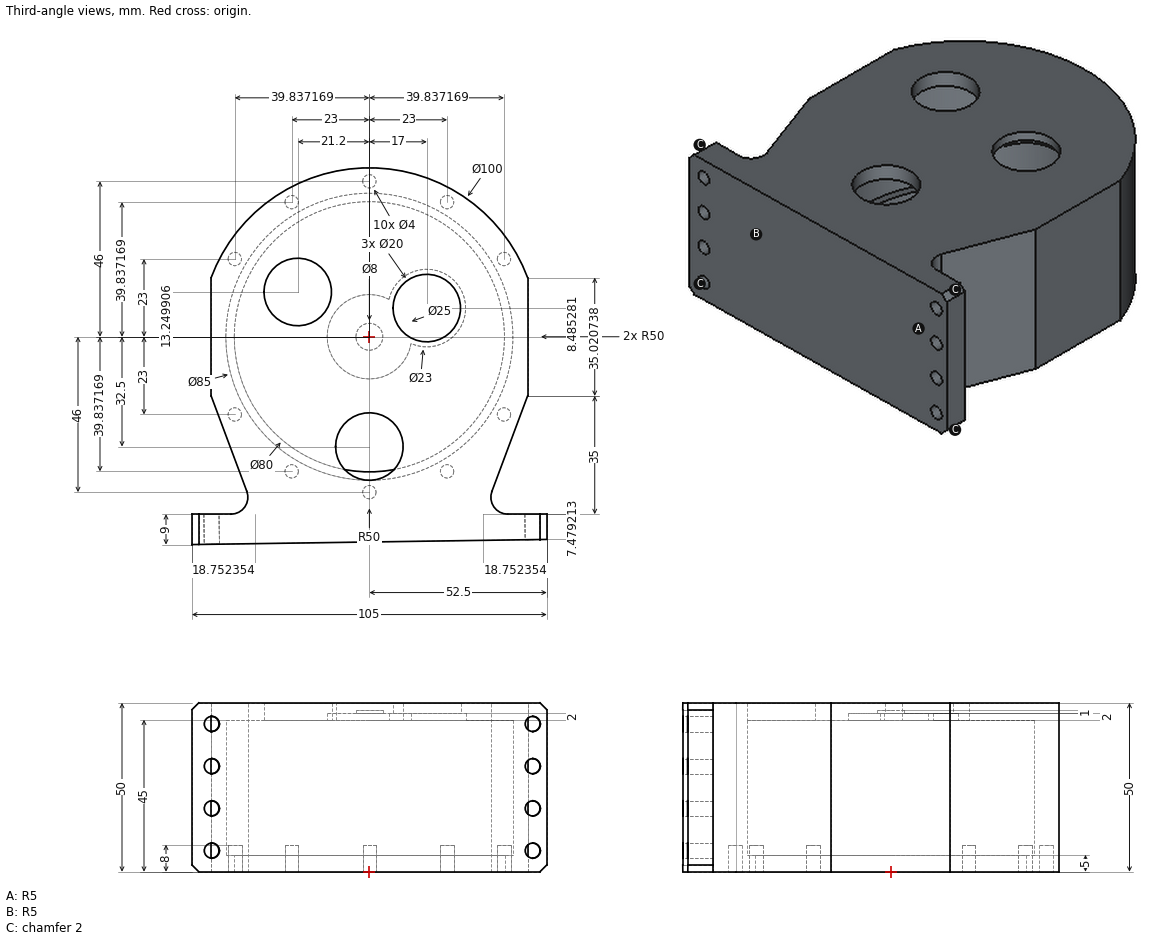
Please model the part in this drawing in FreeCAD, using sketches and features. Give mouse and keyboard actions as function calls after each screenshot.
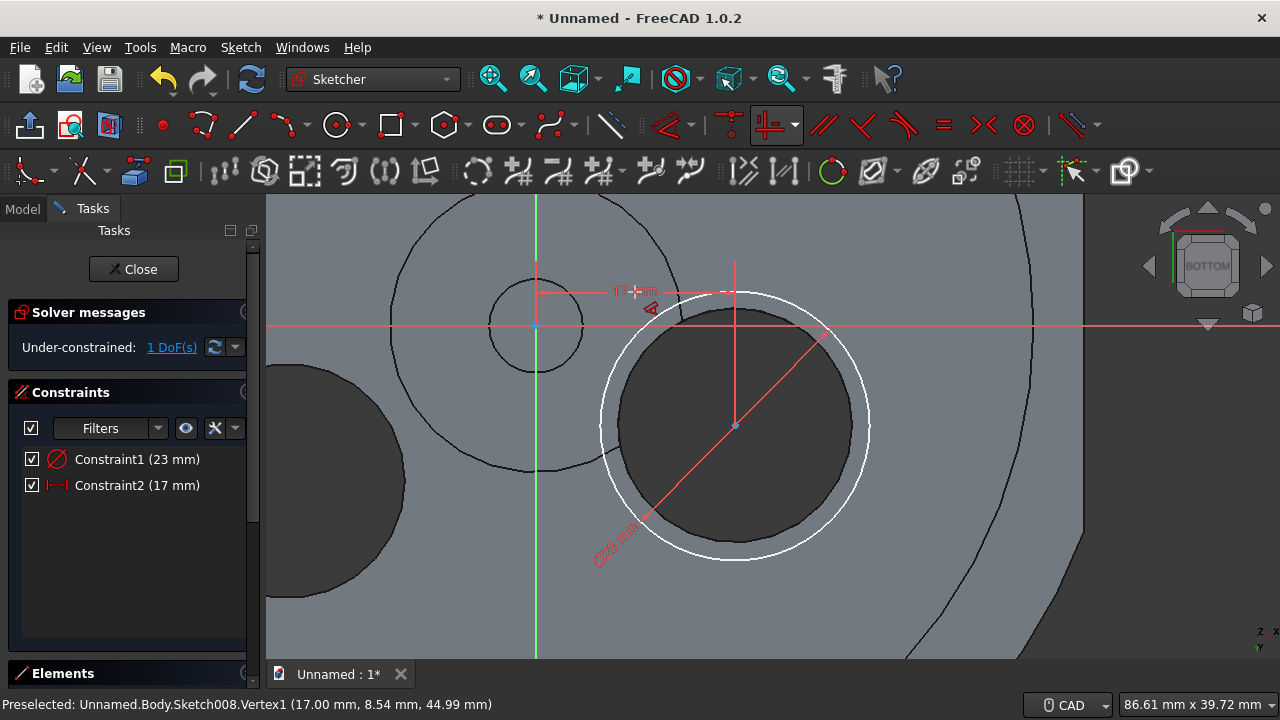
click(735, 426)
click(502, 376)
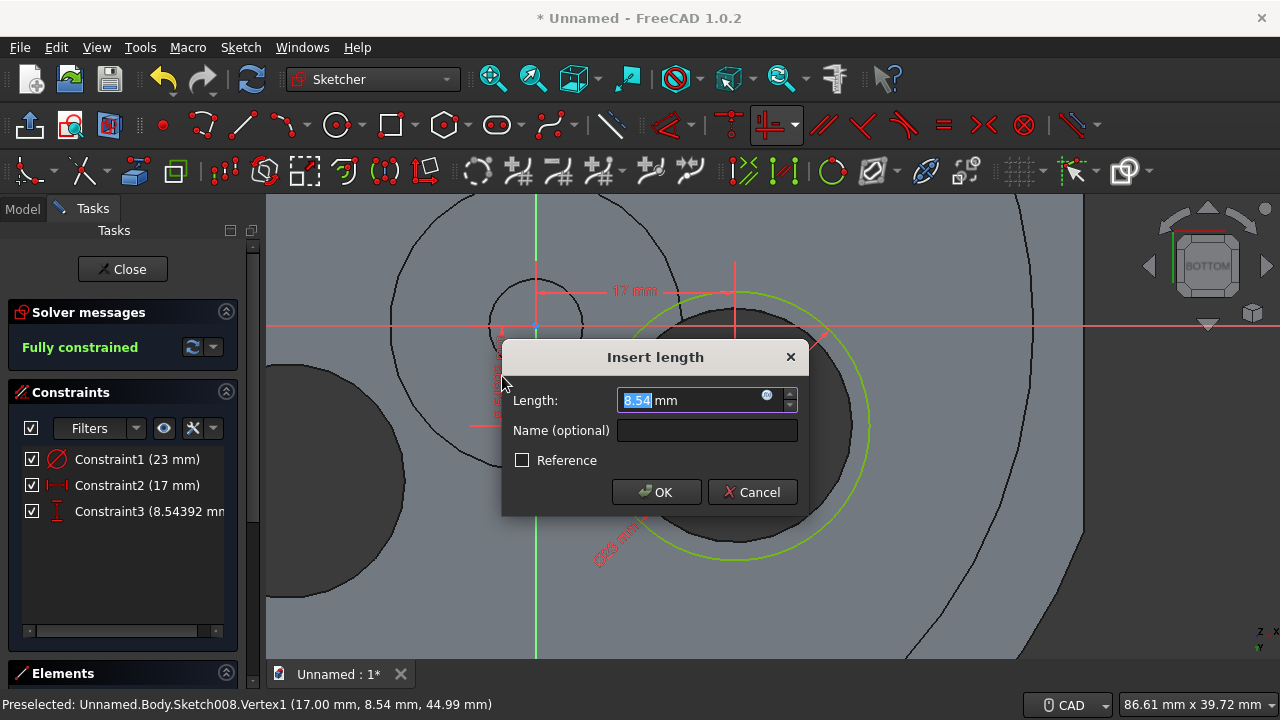
text(8.485281)
key(Return)
key(Escape)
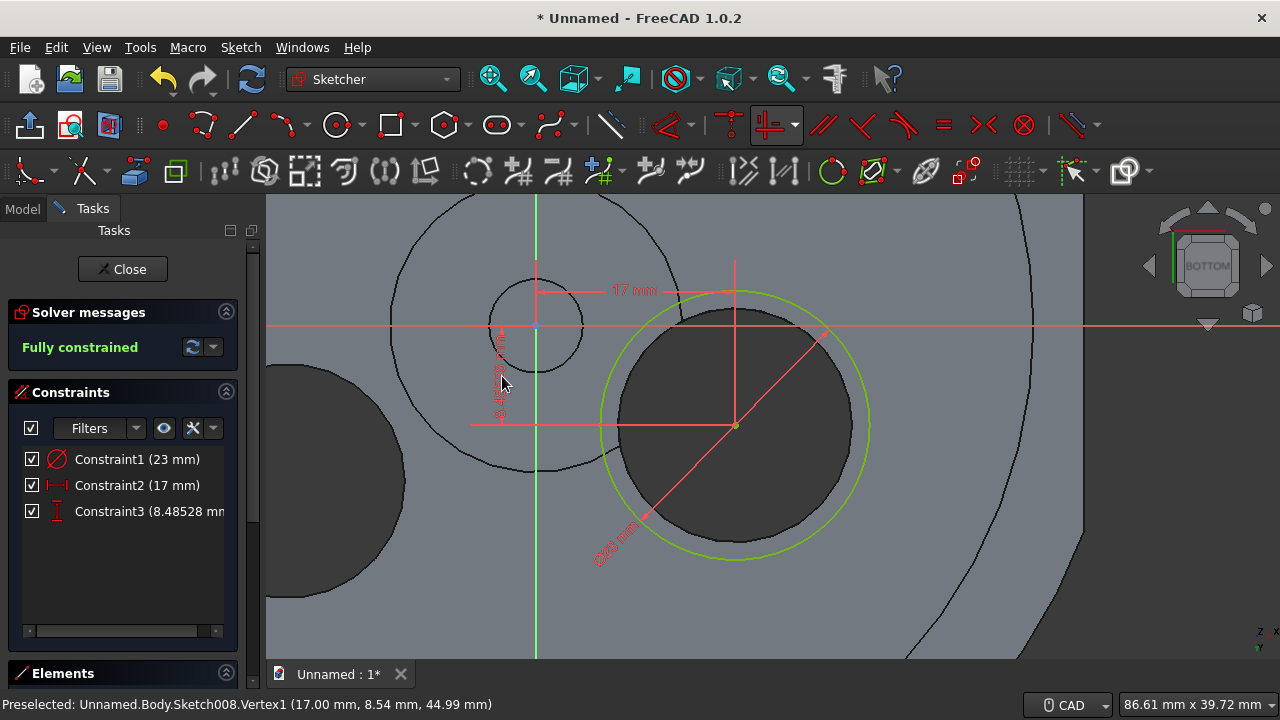
click(123, 269)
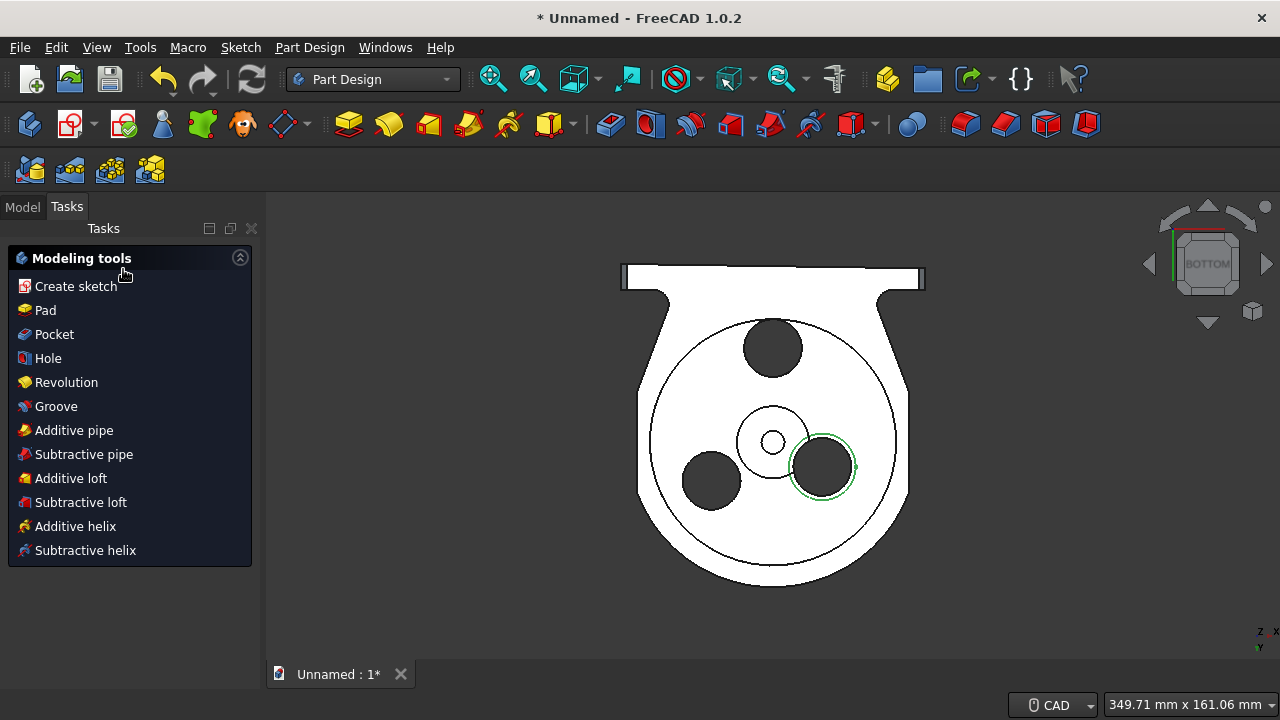
click(612, 124)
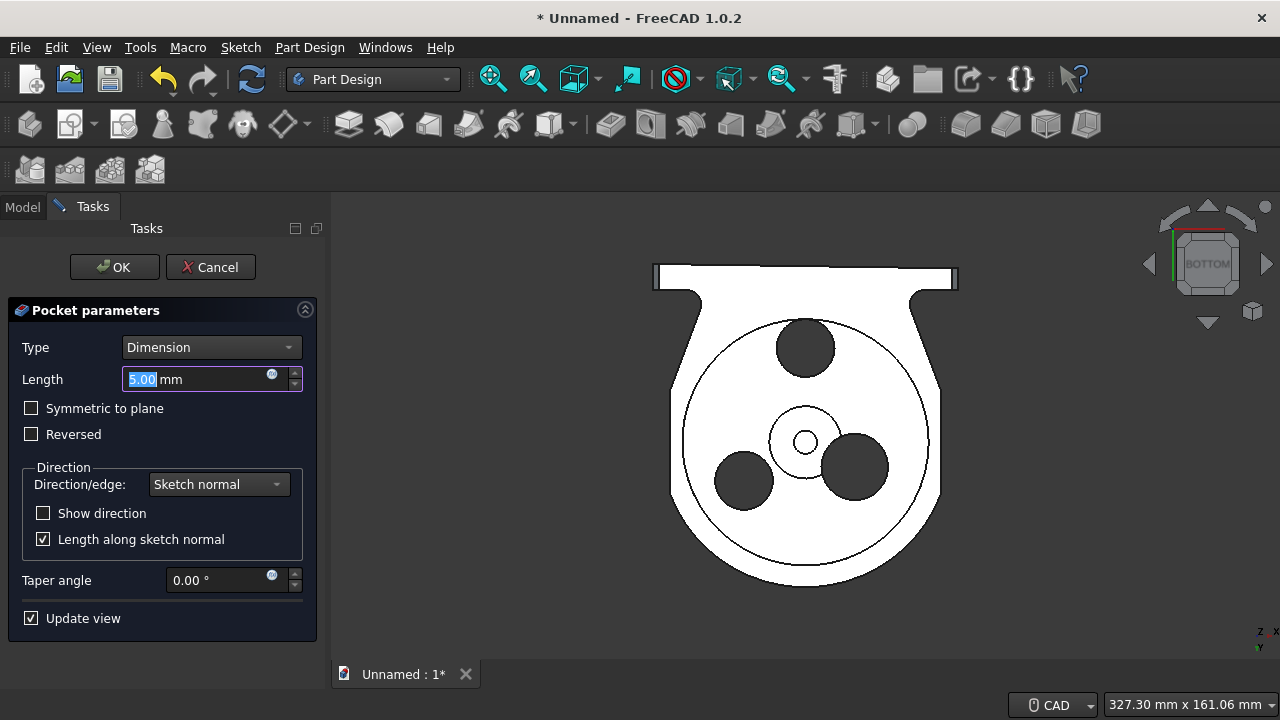
text(2)
key(Tab)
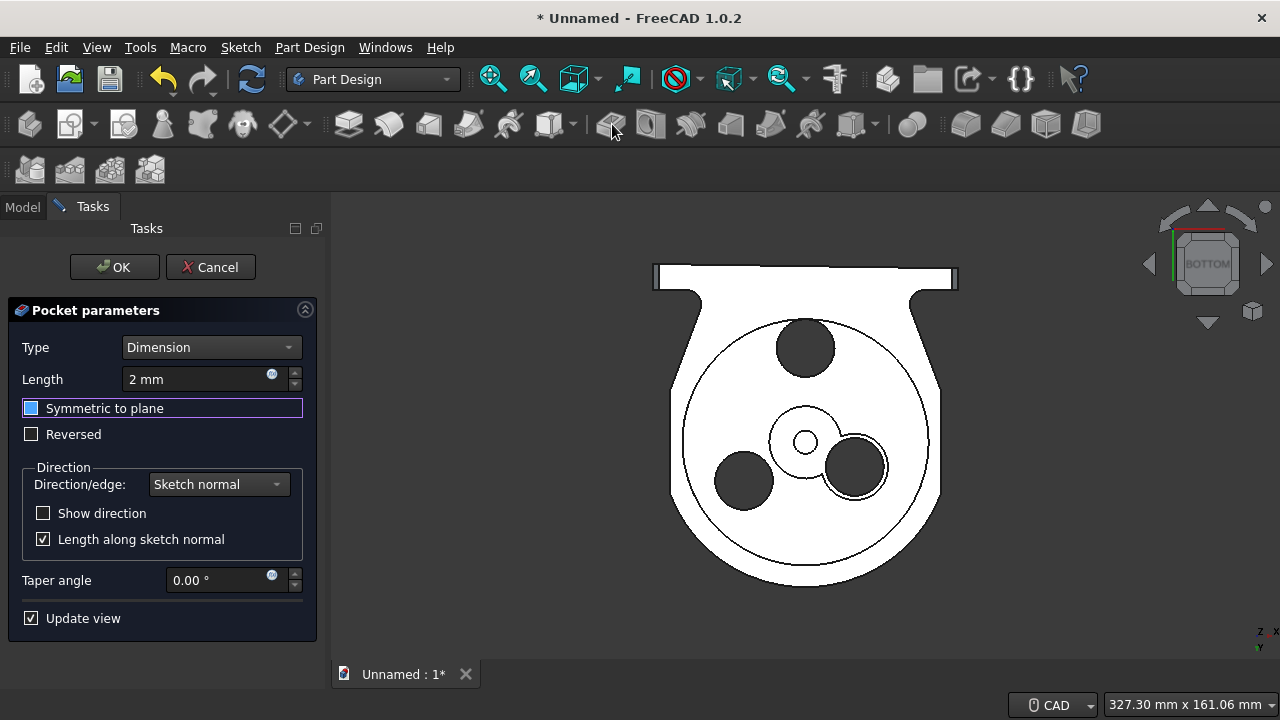
click(115, 267)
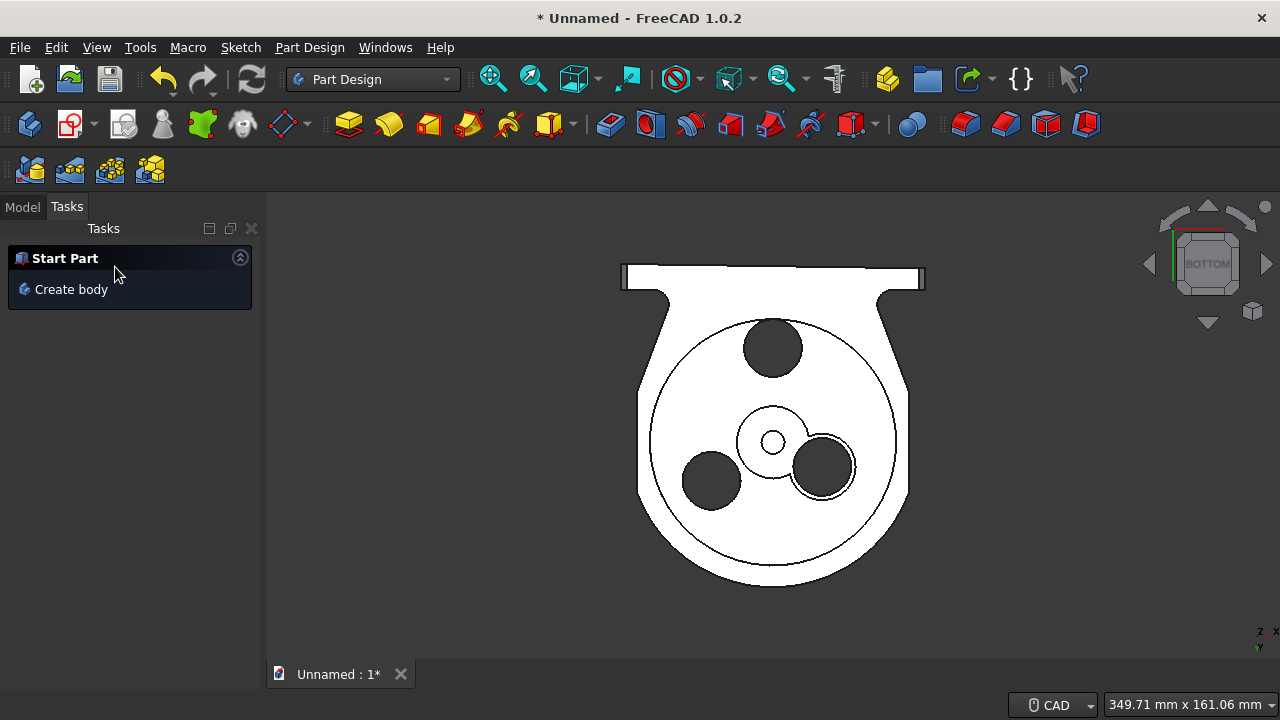
click(70, 124)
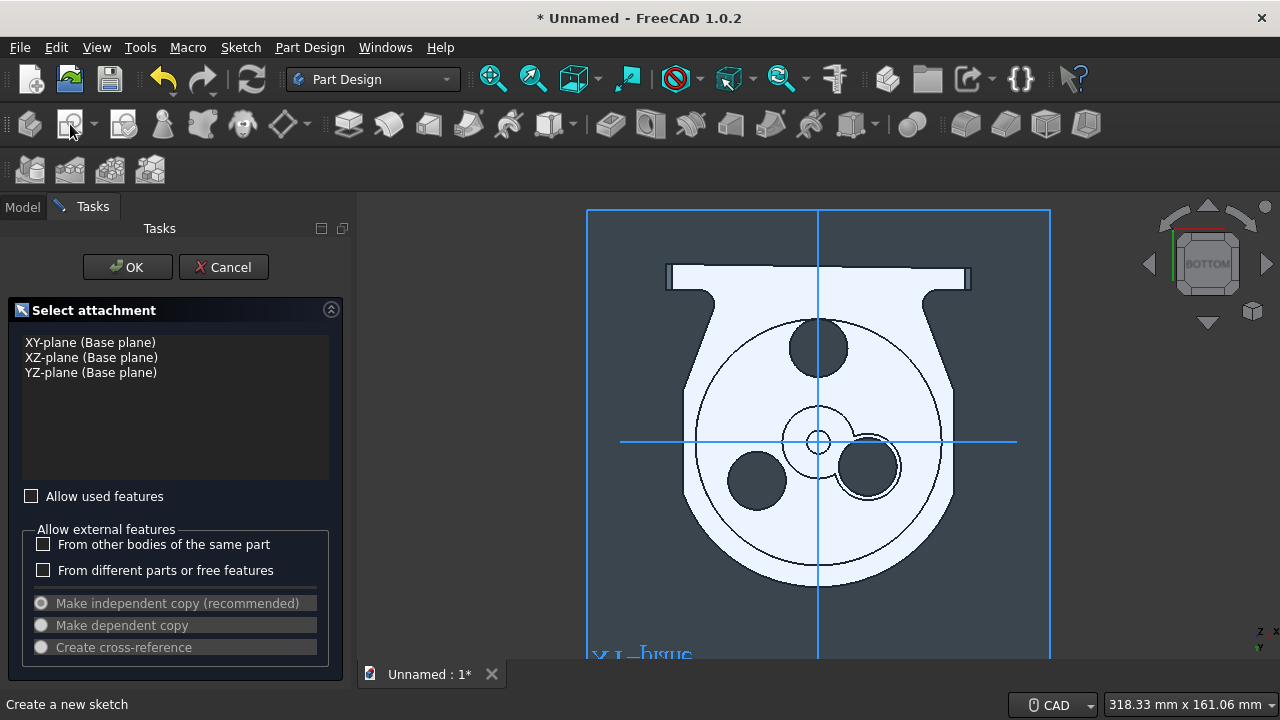
click(82, 342)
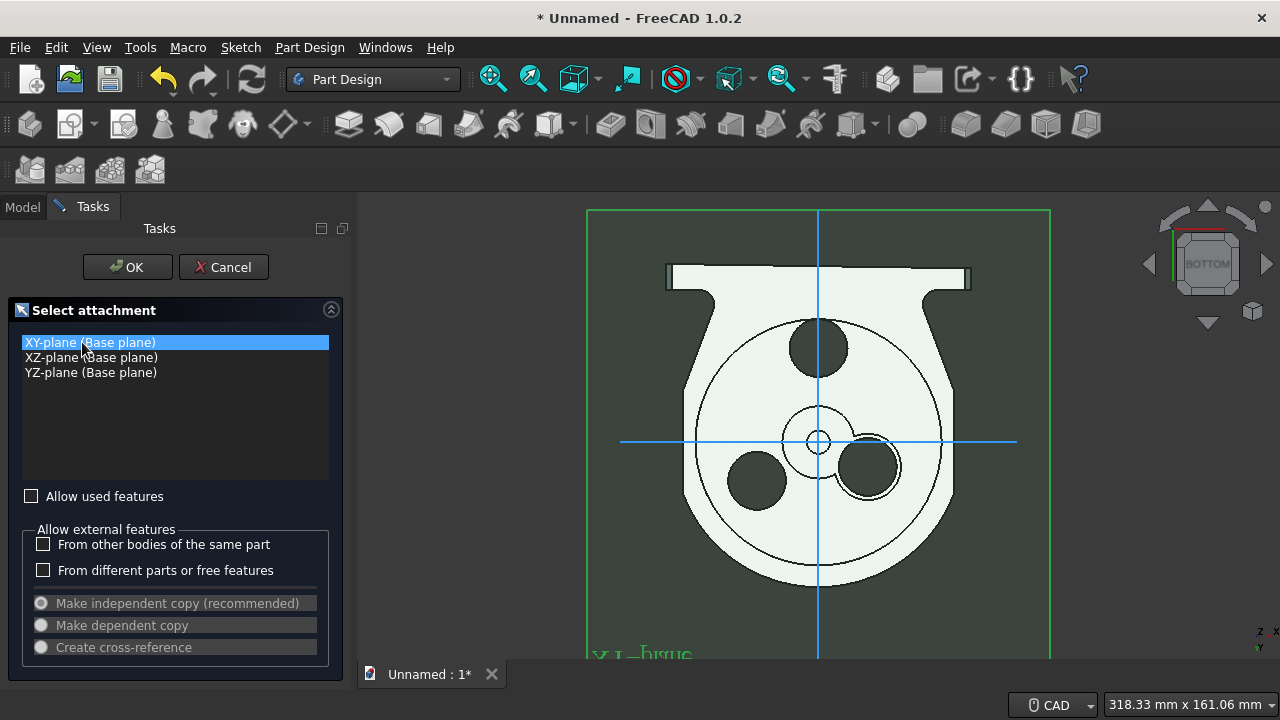
click(128, 267)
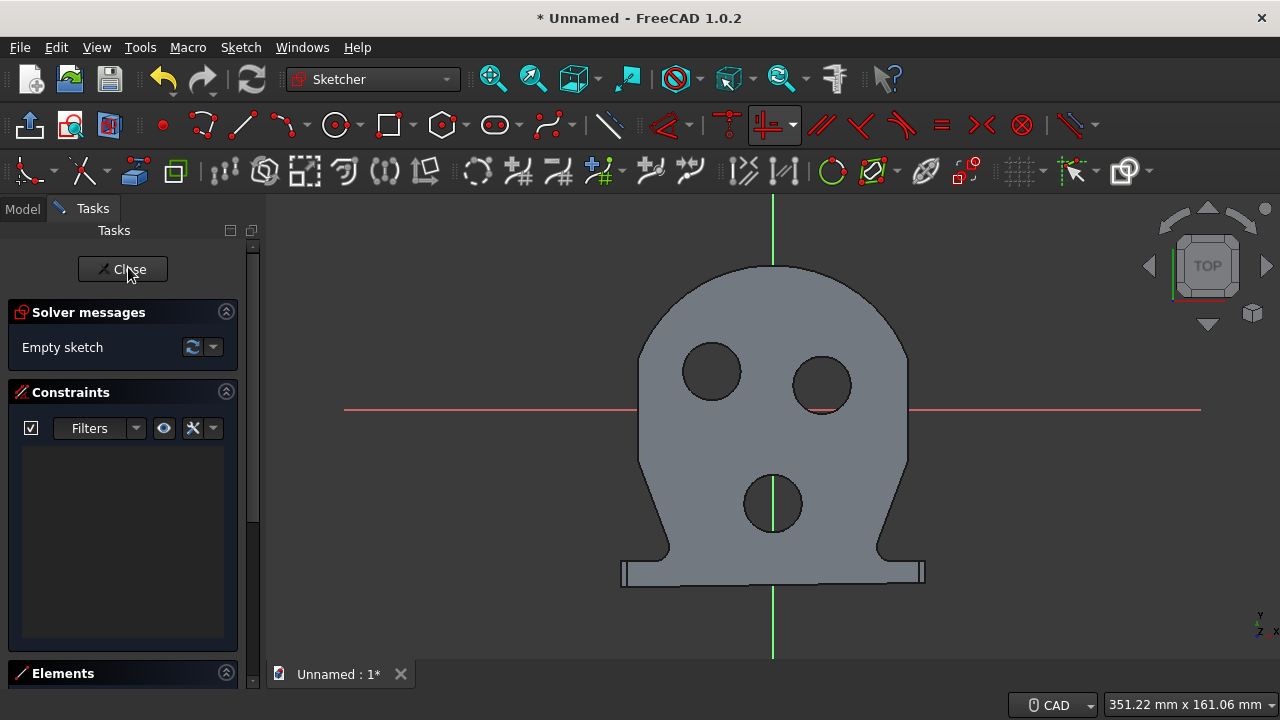
key(q)
key(s)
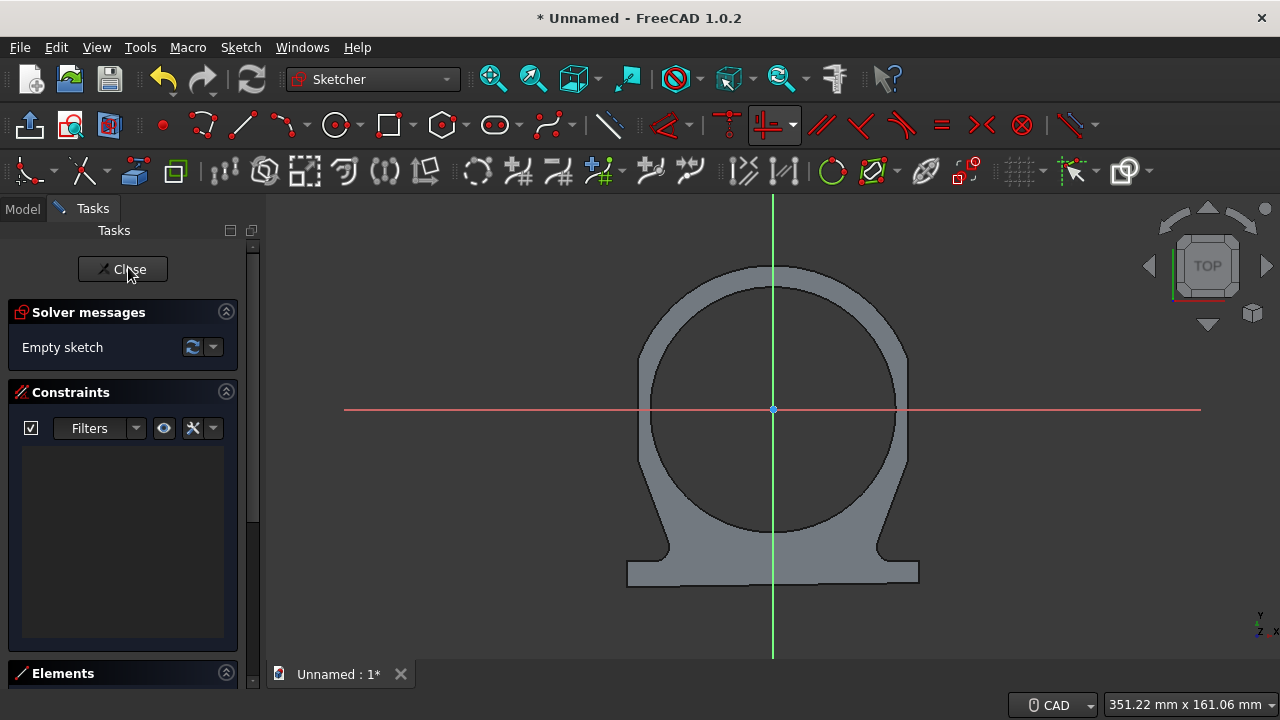
click(336, 126)